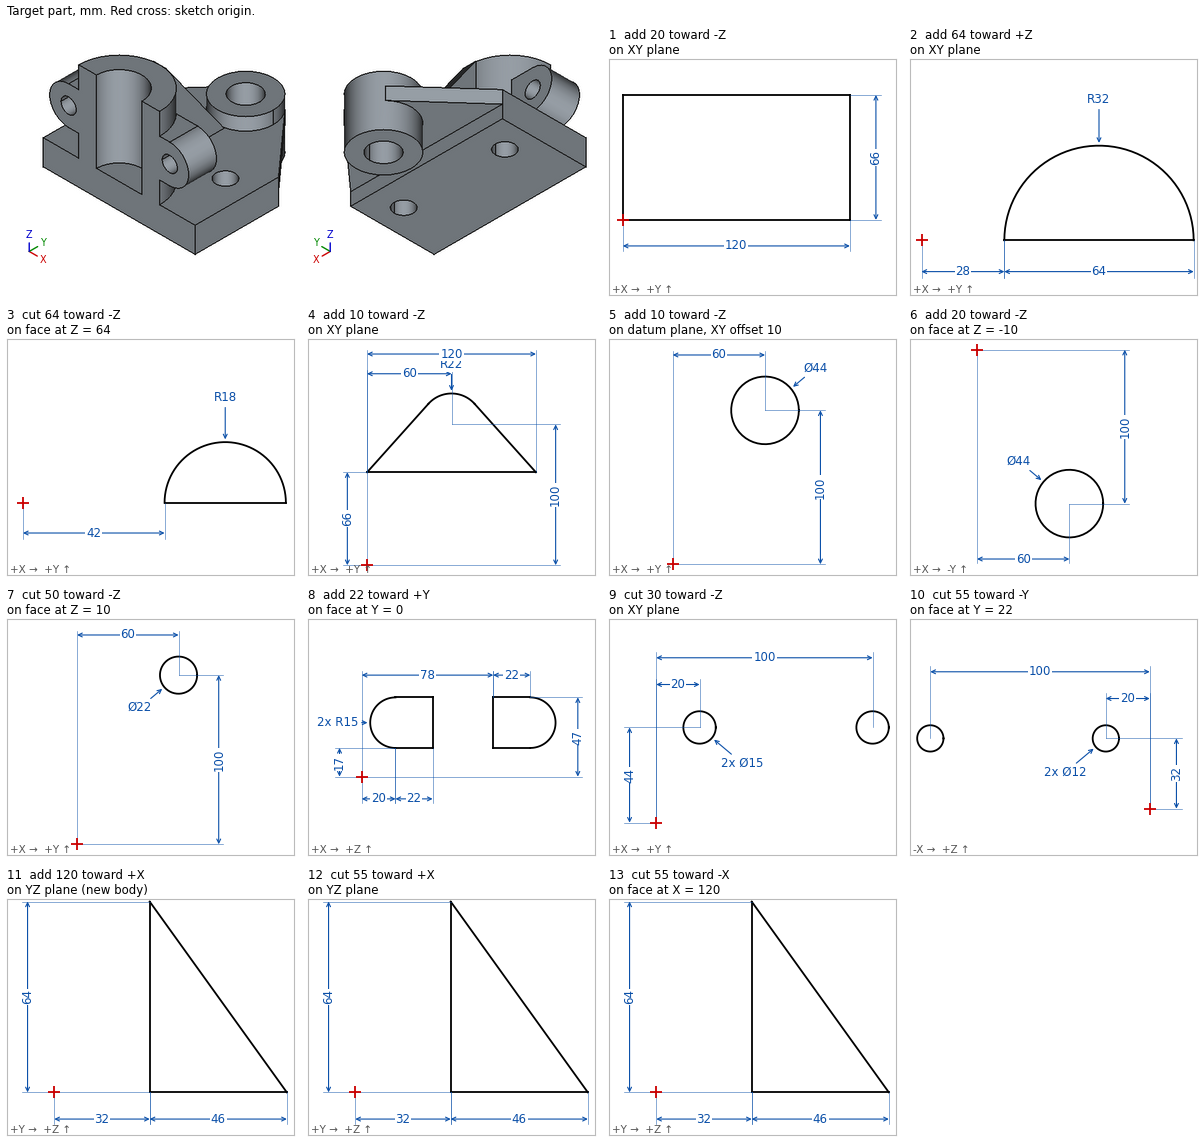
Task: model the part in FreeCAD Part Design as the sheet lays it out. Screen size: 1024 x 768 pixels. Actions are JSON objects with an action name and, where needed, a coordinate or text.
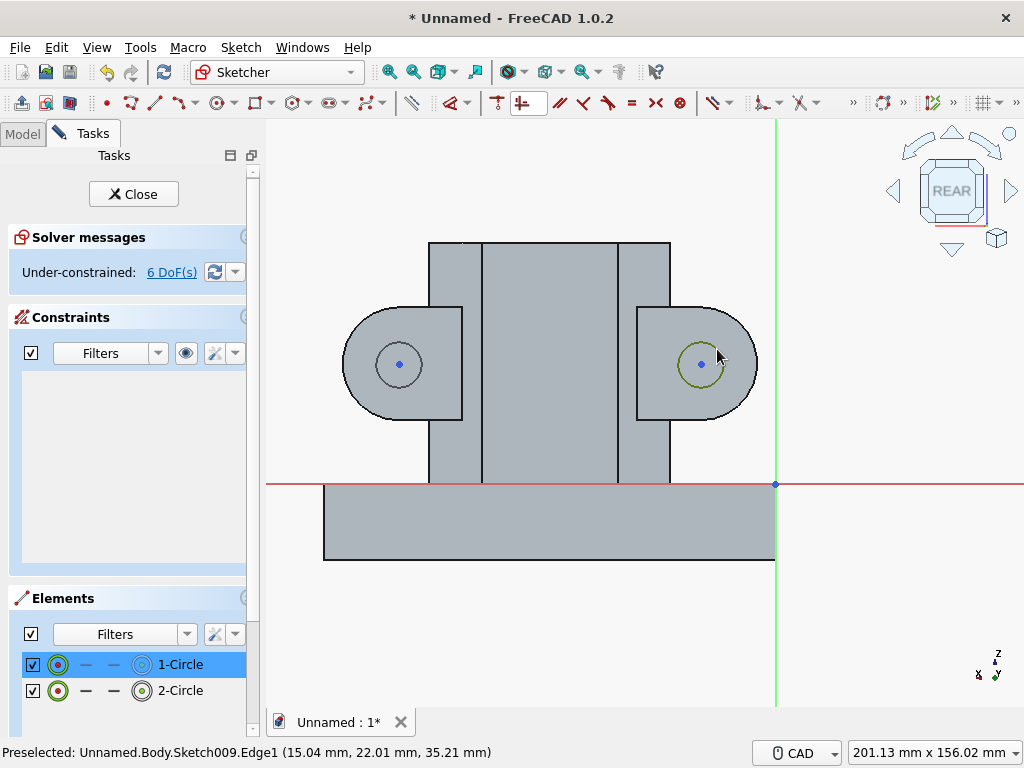
{"action": "left_click", "coordinate": [415, 349]}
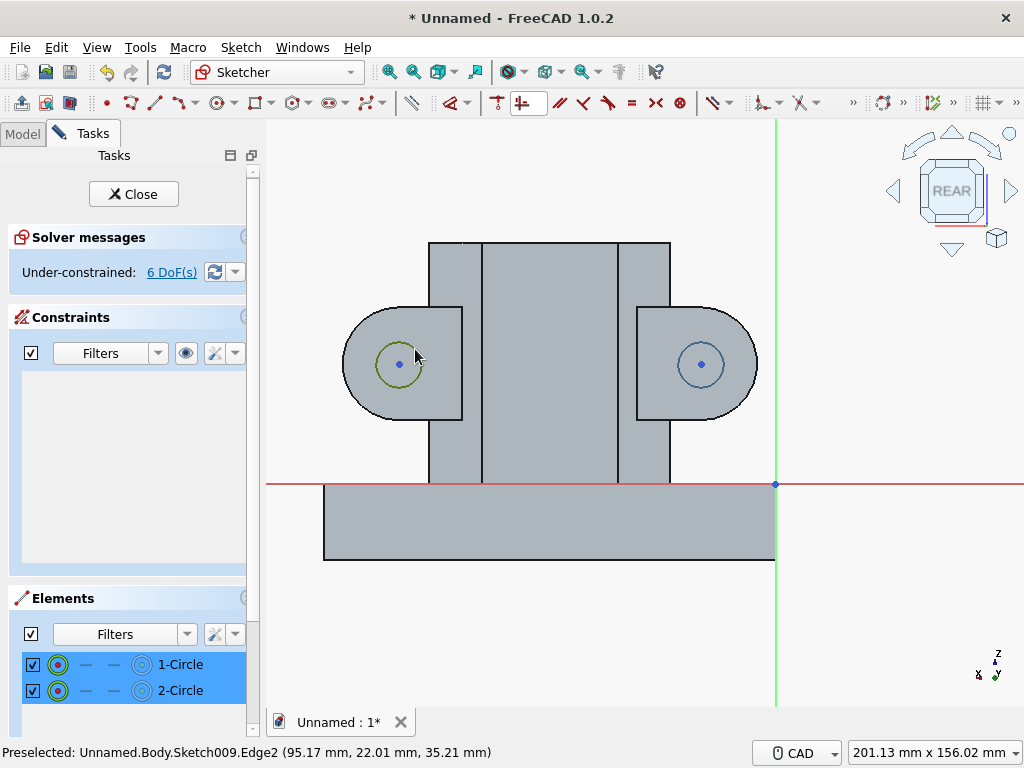
{"action": "left_click", "coordinate": [632, 104]}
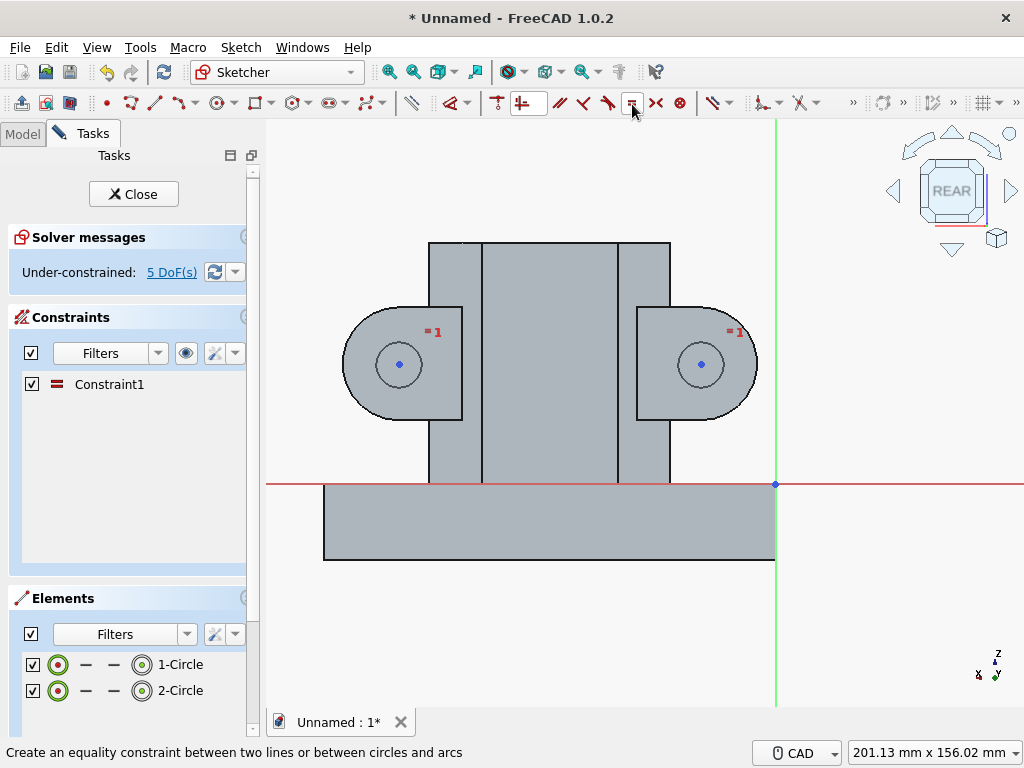
{"action": "left_click", "coordinate": [701, 365]}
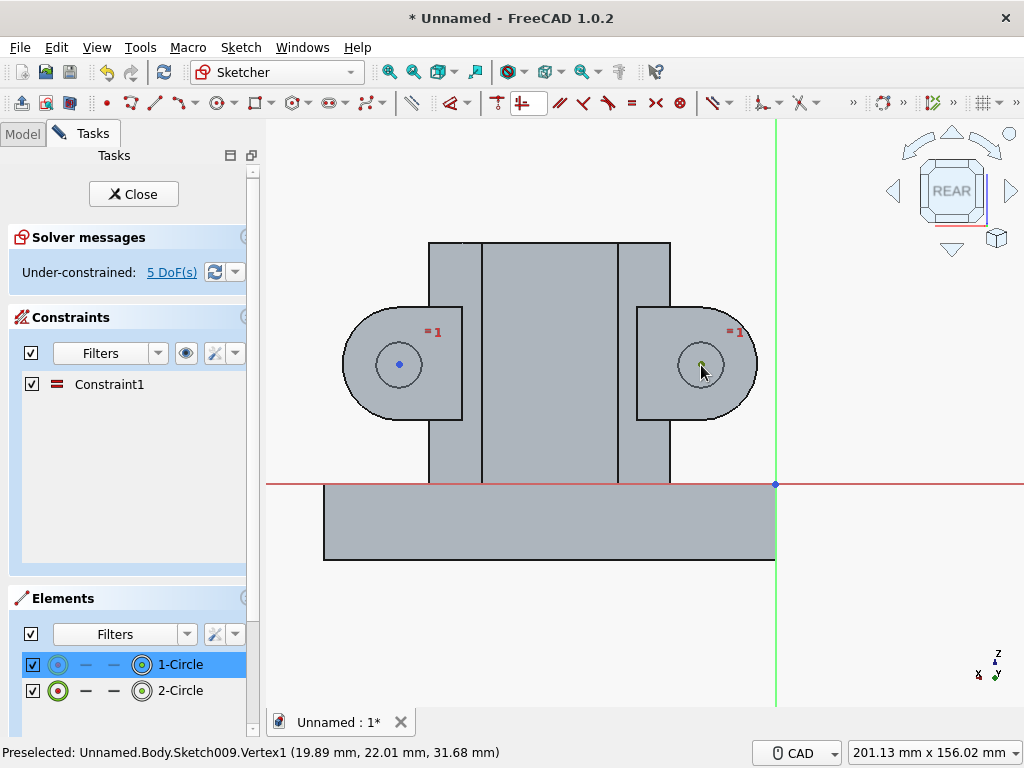
{"action": "left_click", "coordinate": [399, 365]}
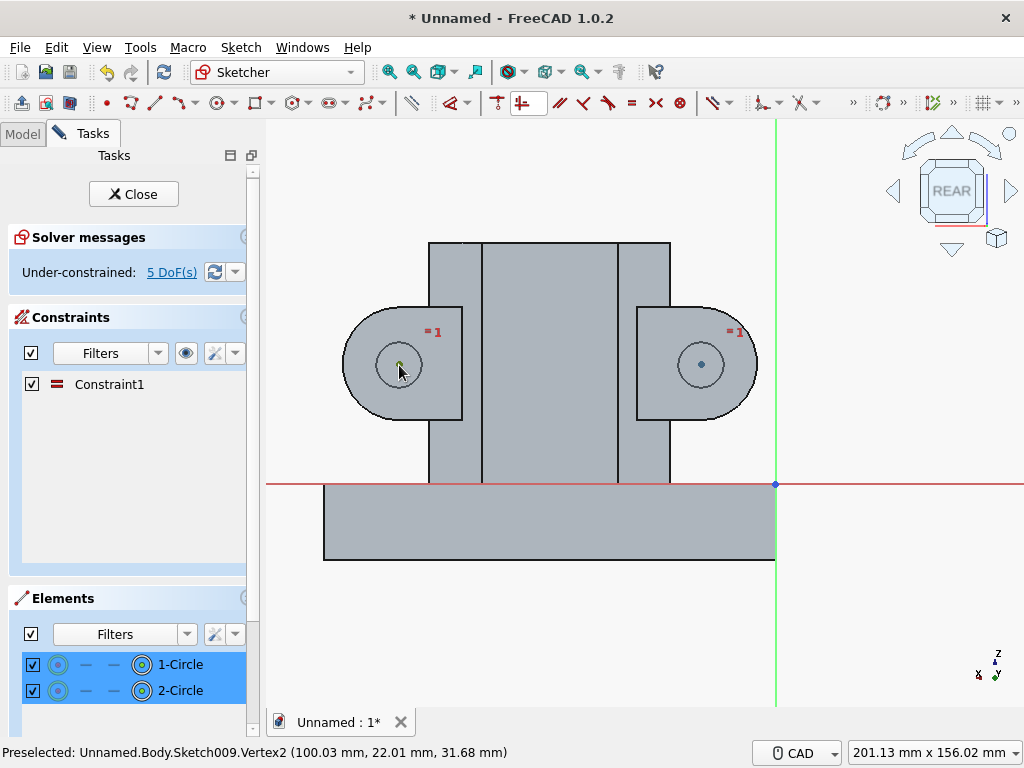
{"action": "left_click", "coordinate": [542, 104]}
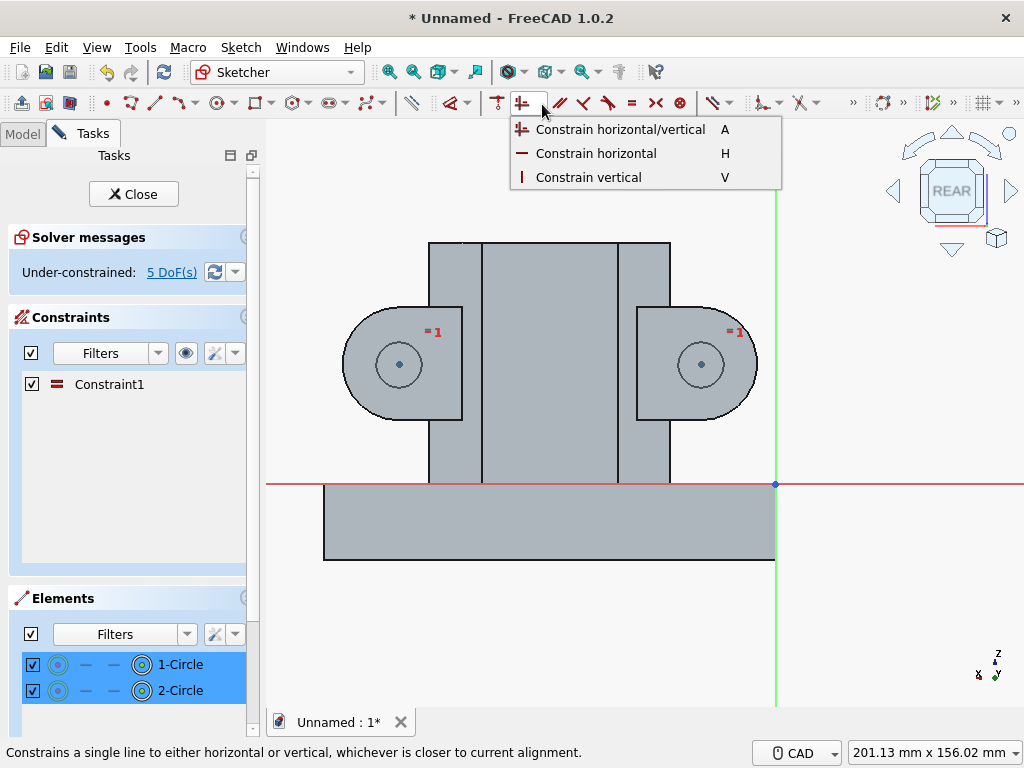
{"action": "left_click", "coordinate": [646, 153]}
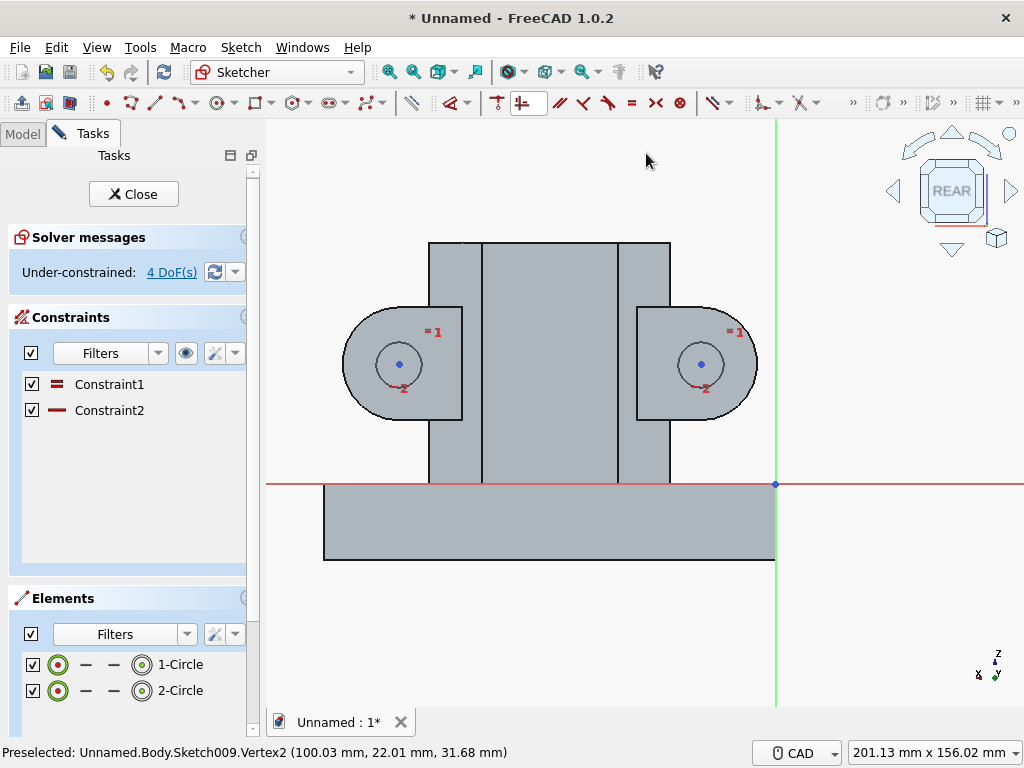
{"action": "left_click", "coordinate": [450, 104]}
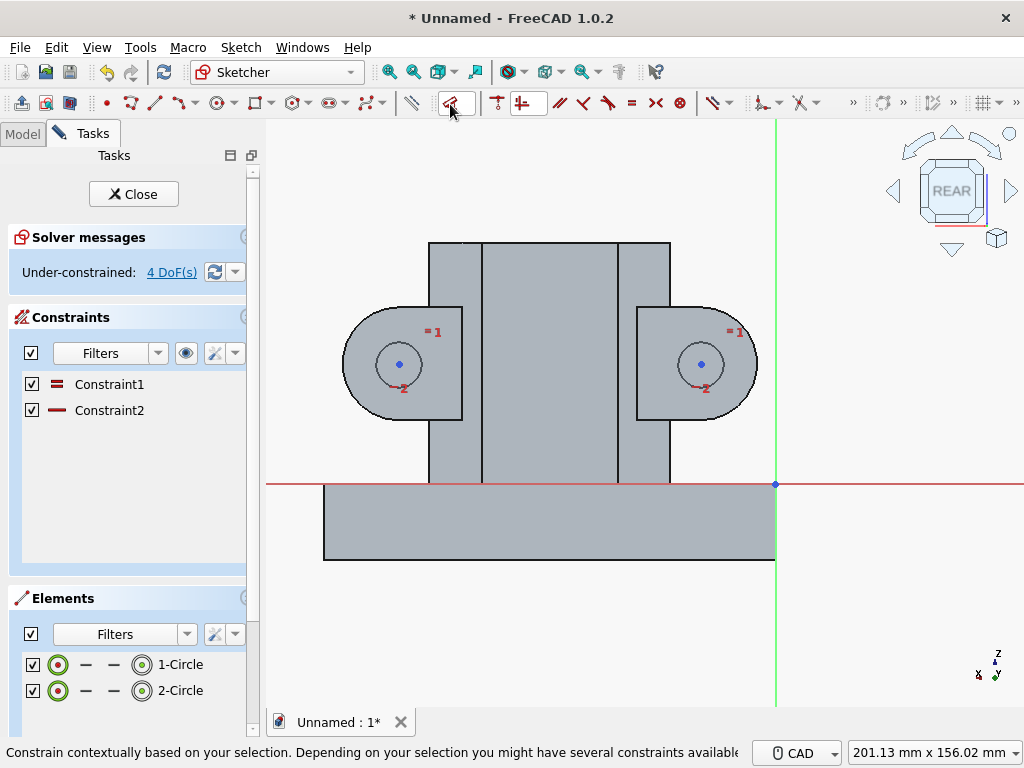
{"action": "left_click", "coordinate": [717, 349]}
{"action": "left_click", "coordinate": [740, 326]}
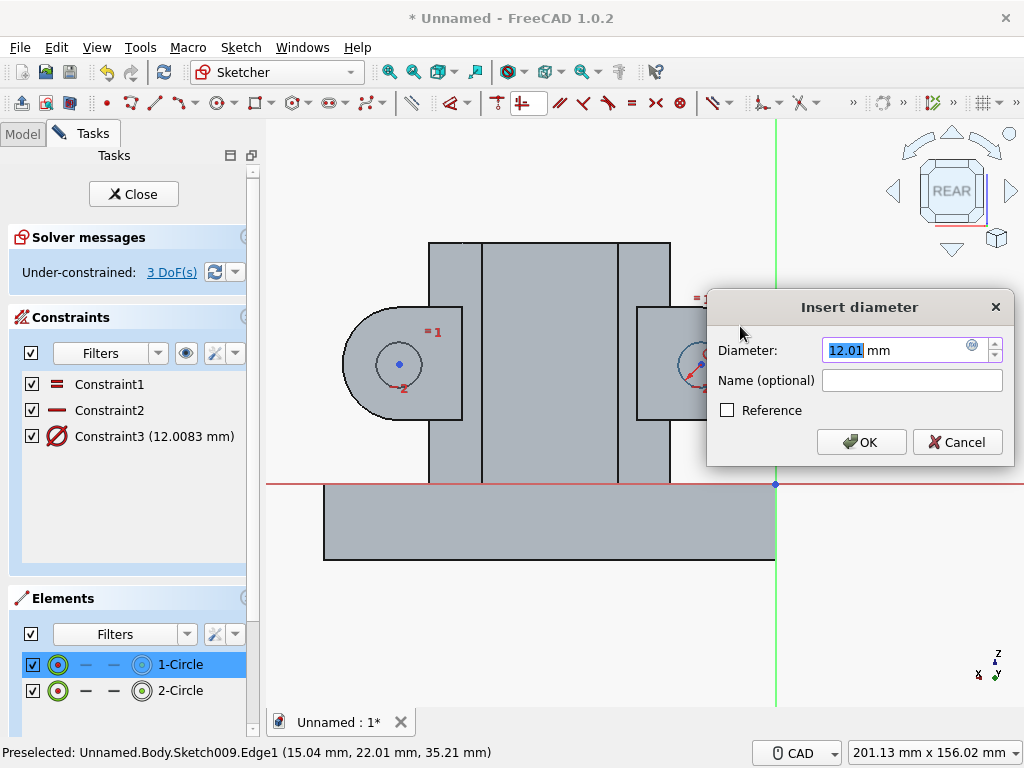
{"action": "type", "text": "12"}
{"action": "key", "text": "Return"}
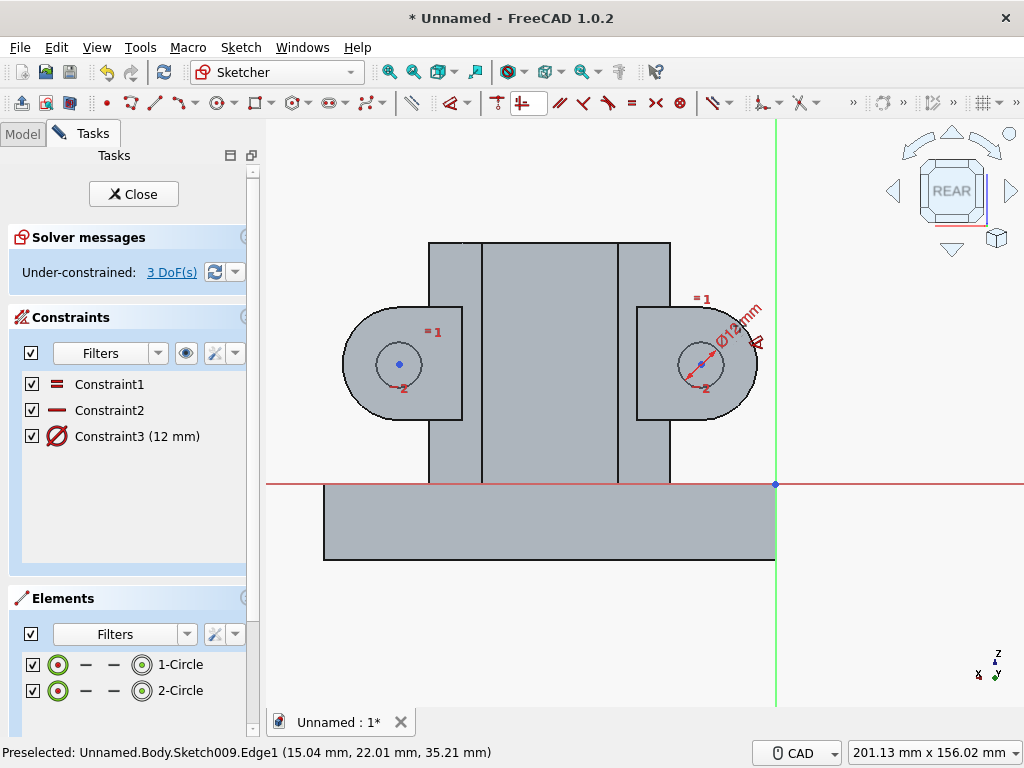
{"action": "left_click", "coordinate": [701, 365]}
{"action": "left_click", "coordinate": [738, 518]}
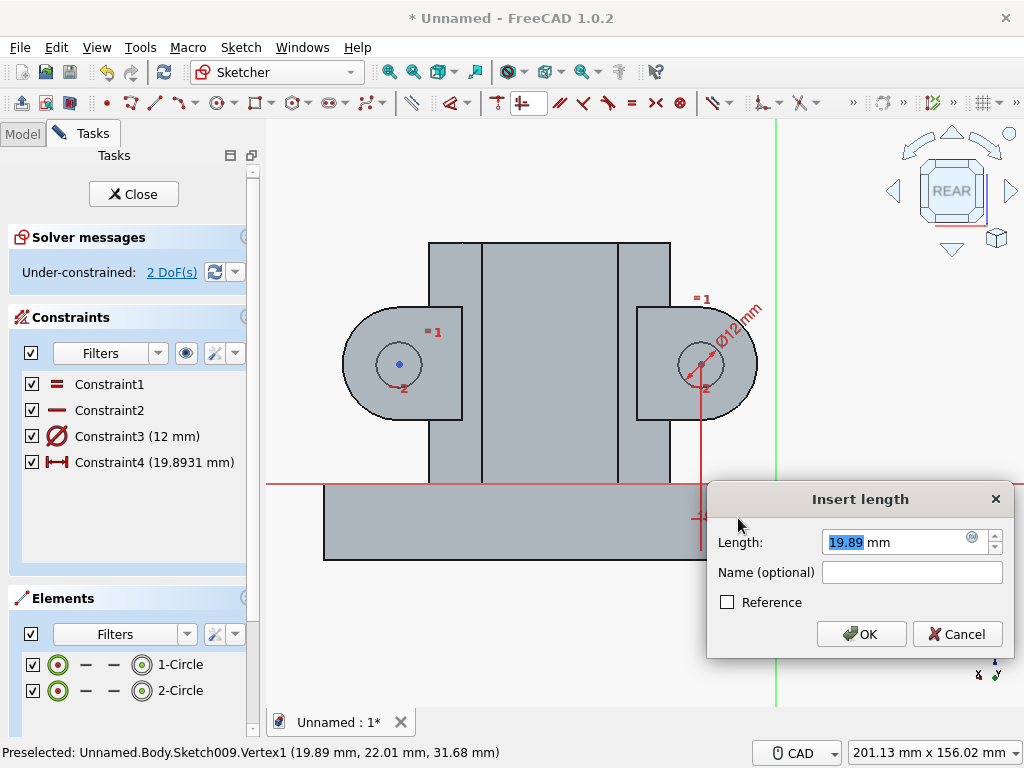
{"action": "type", "text": "20"}
{"action": "key", "text": "Return"}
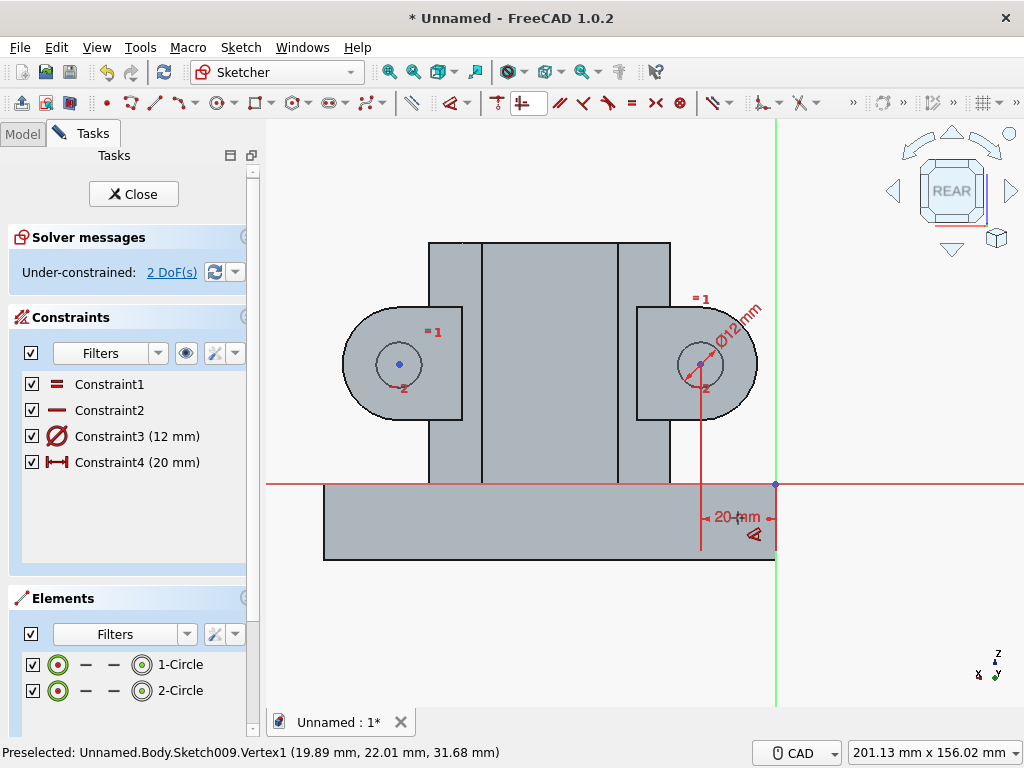
{"action": "left_click", "coordinate": [701, 365]}
{"action": "left_click", "coordinate": [810, 425]}